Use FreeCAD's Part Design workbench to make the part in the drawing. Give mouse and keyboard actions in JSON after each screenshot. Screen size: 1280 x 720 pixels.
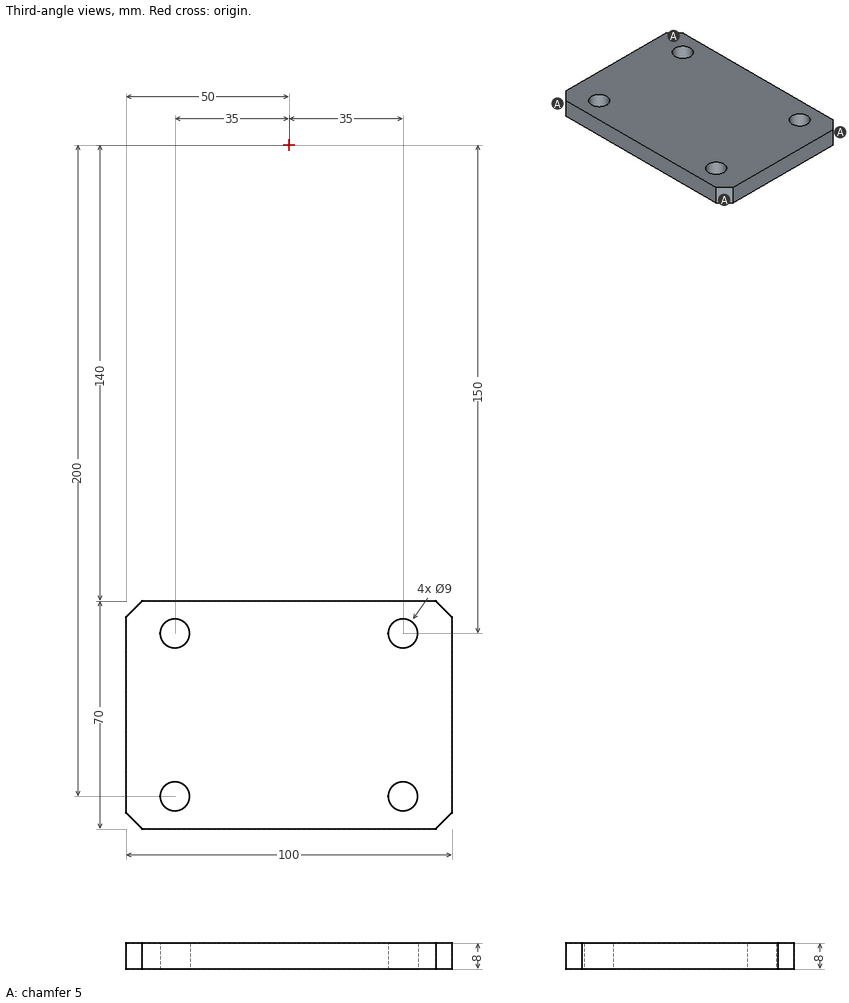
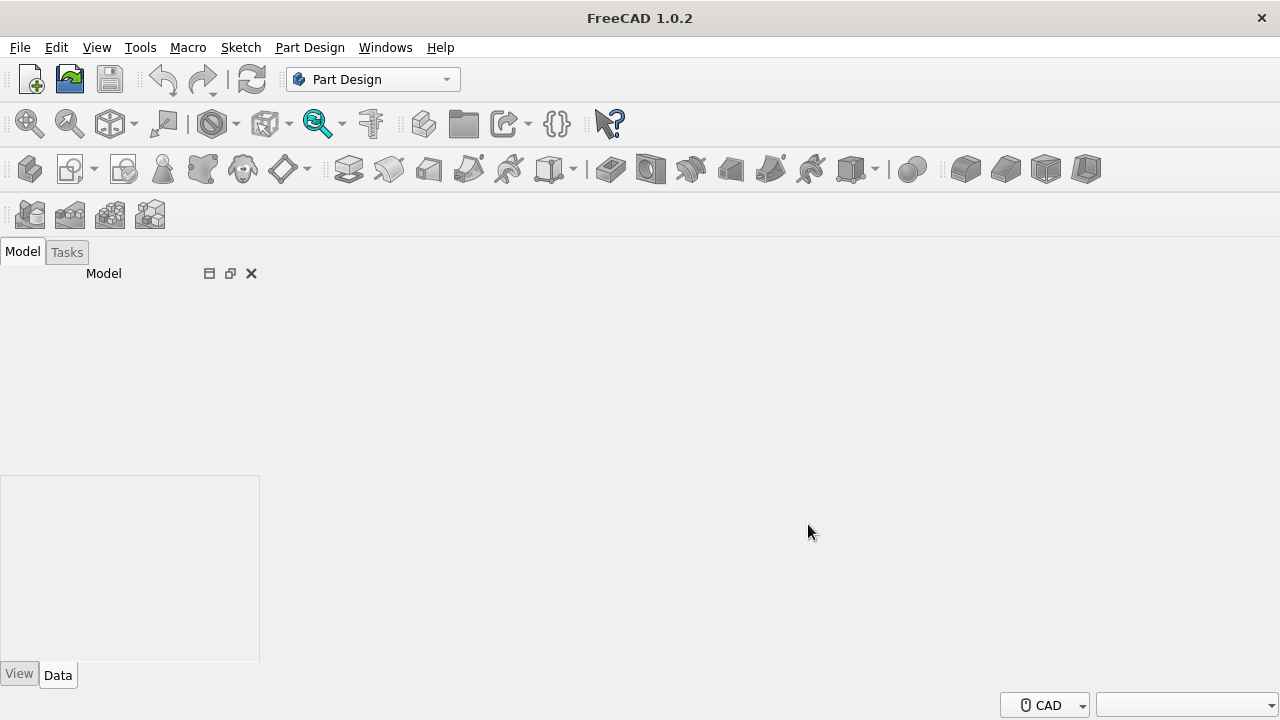
{"action": "left_click", "coordinate": [30, 80]}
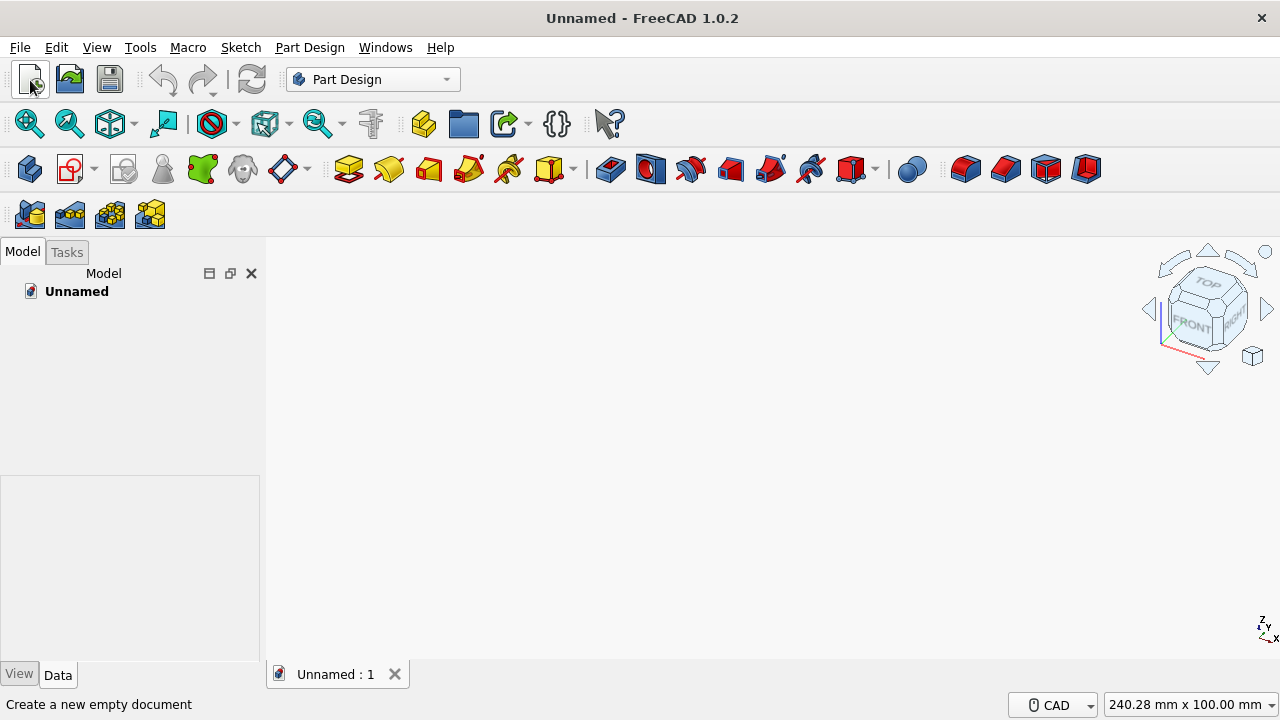
{"action": "left_click", "coordinate": [30, 170]}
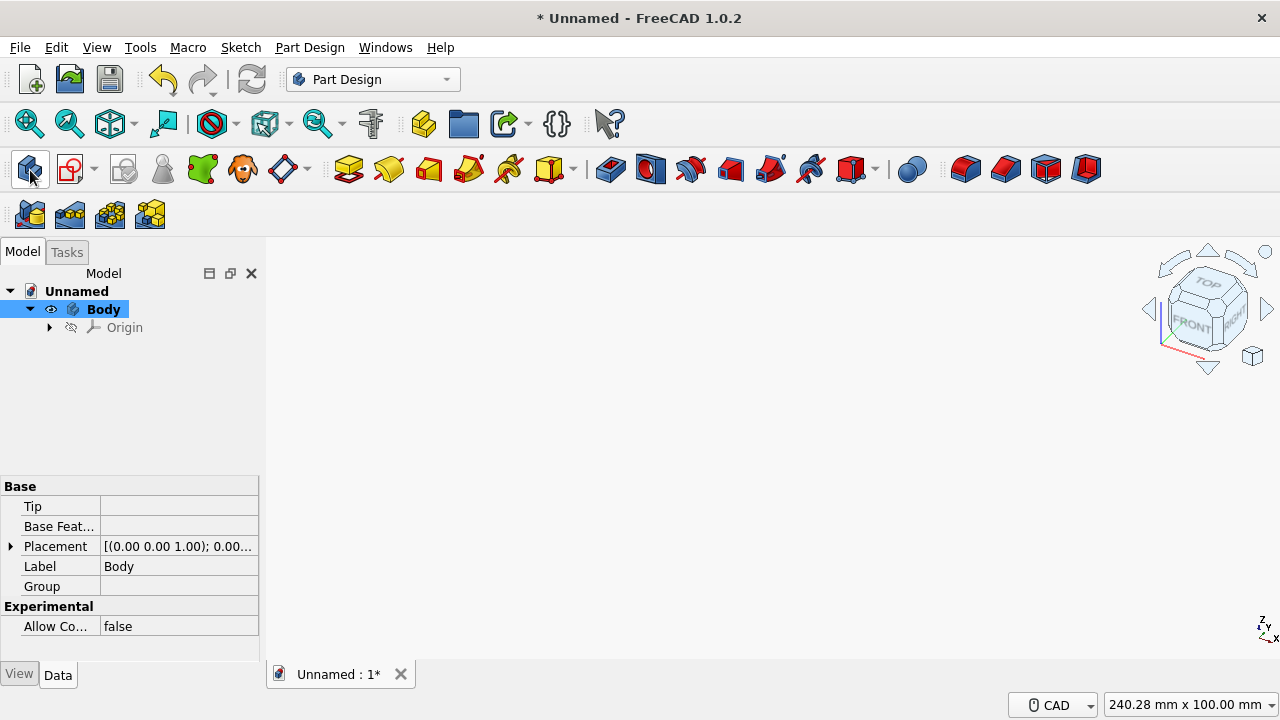
{"action": "left_click", "coordinate": [50, 327]}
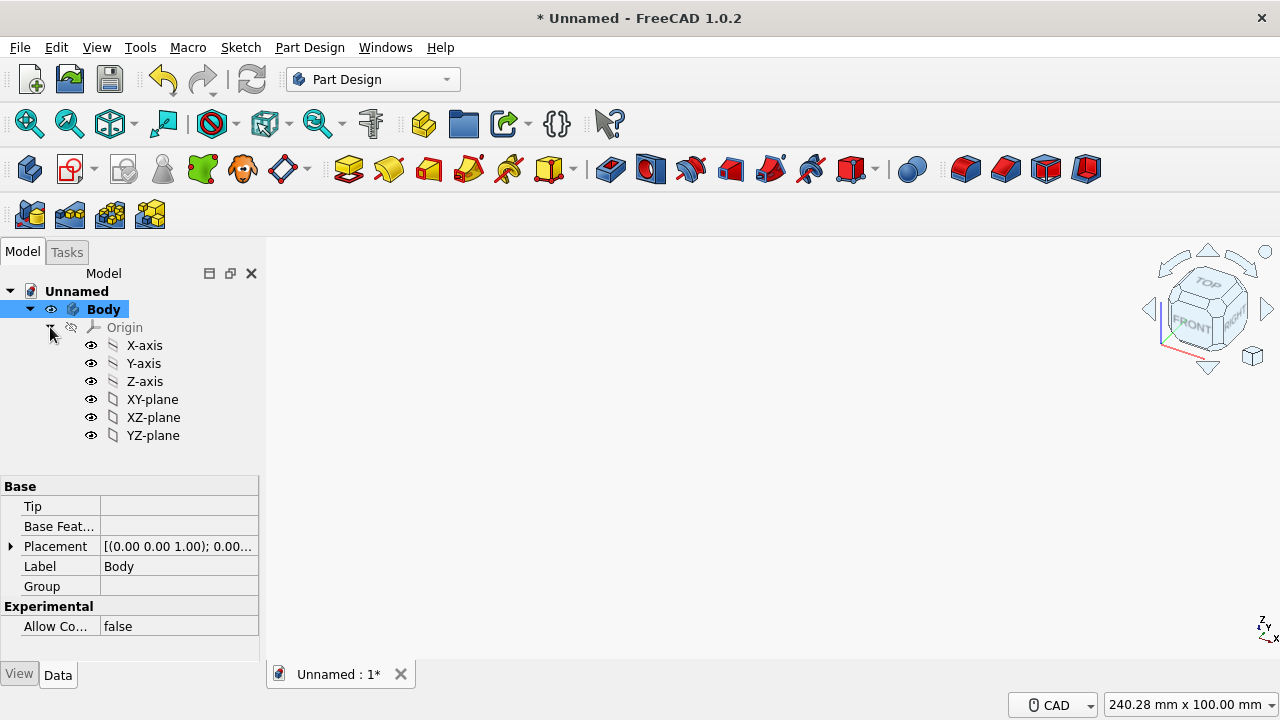
{"action": "left_click", "coordinate": [136, 399]}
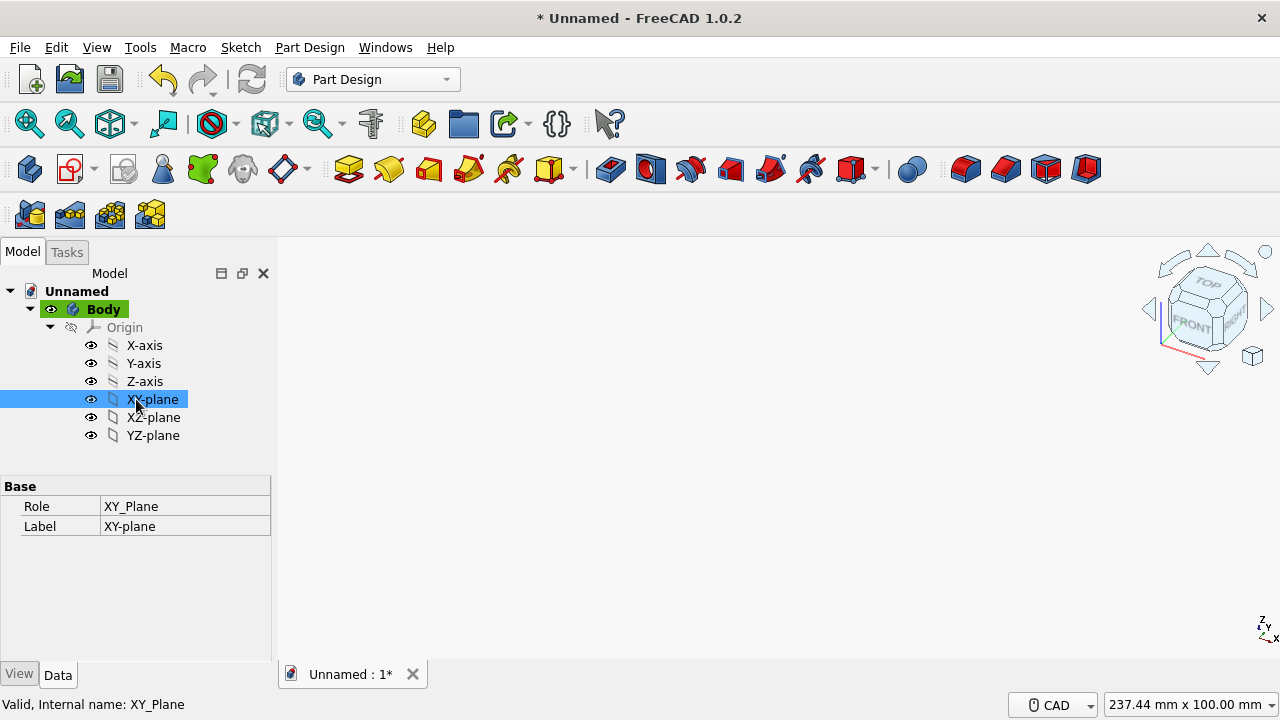
{"action": "left_click", "coordinate": [284, 170]}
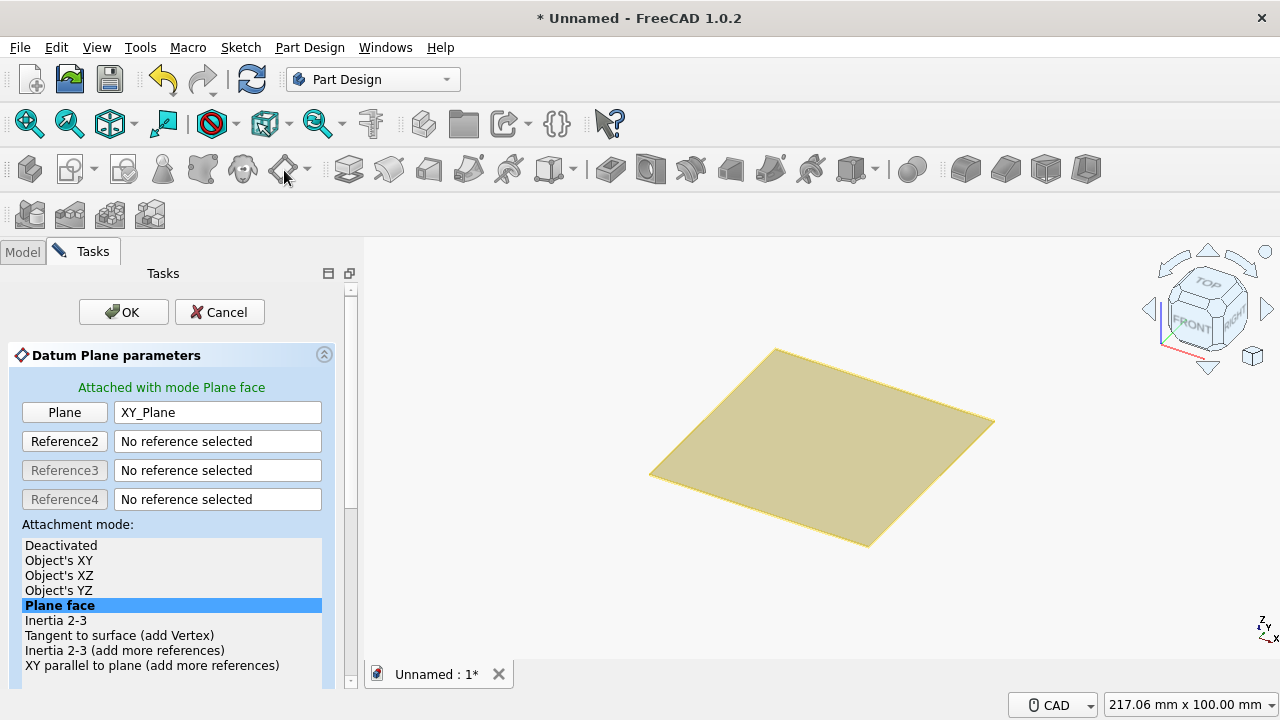
{"action": "scroll", "coordinate": [351, 486], "scroll_direction": "down", "scroll_amount": 4}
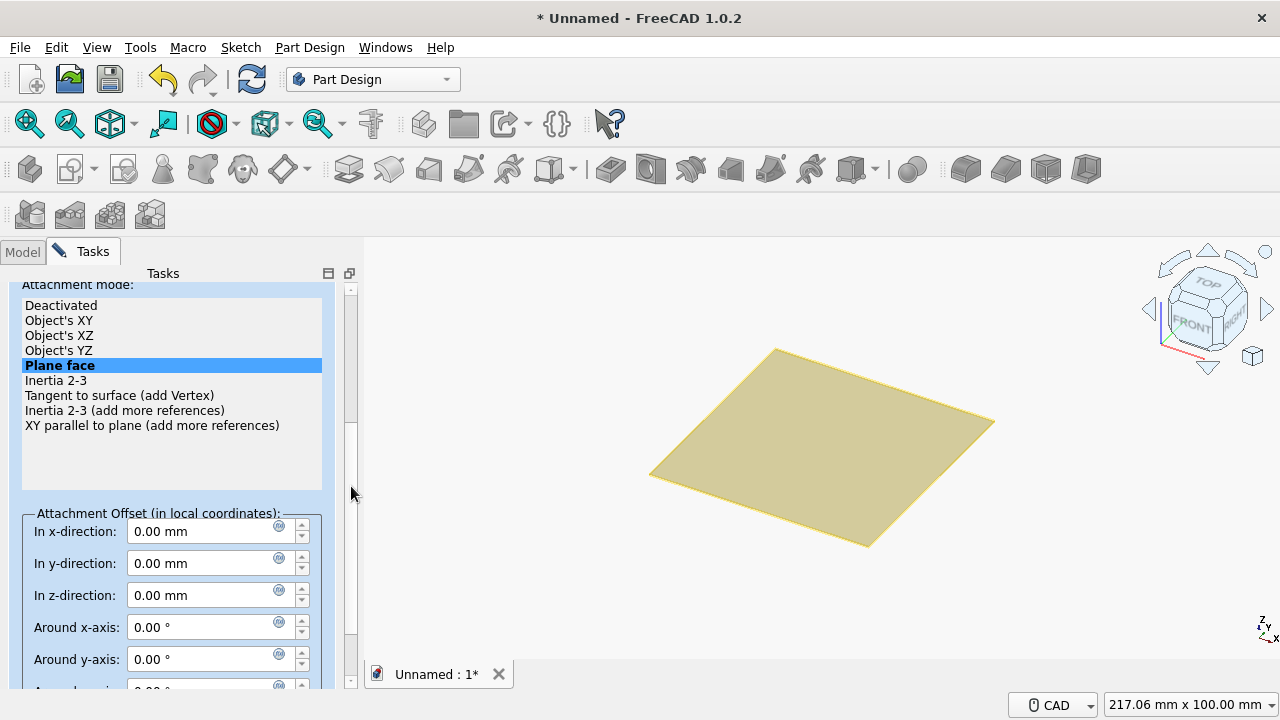
{"action": "triple_click", "coordinate": [210, 595]}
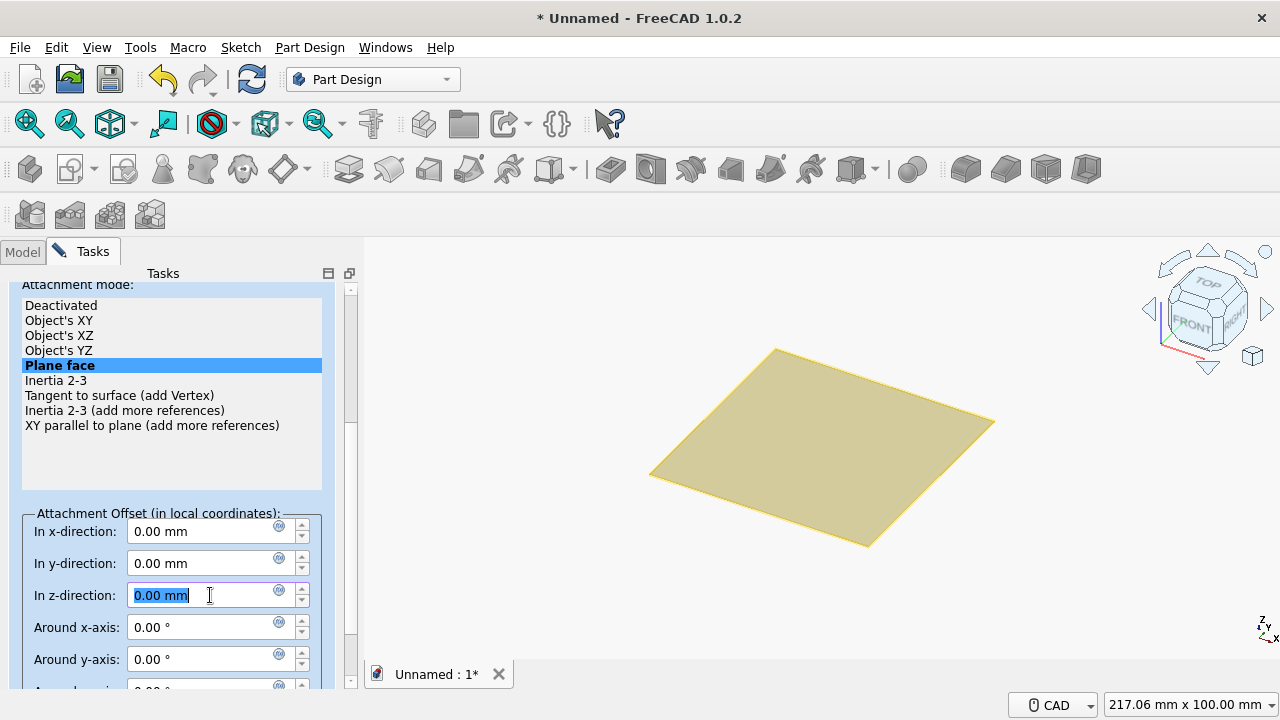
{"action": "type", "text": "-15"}
{"action": "key", "text": "Tab"}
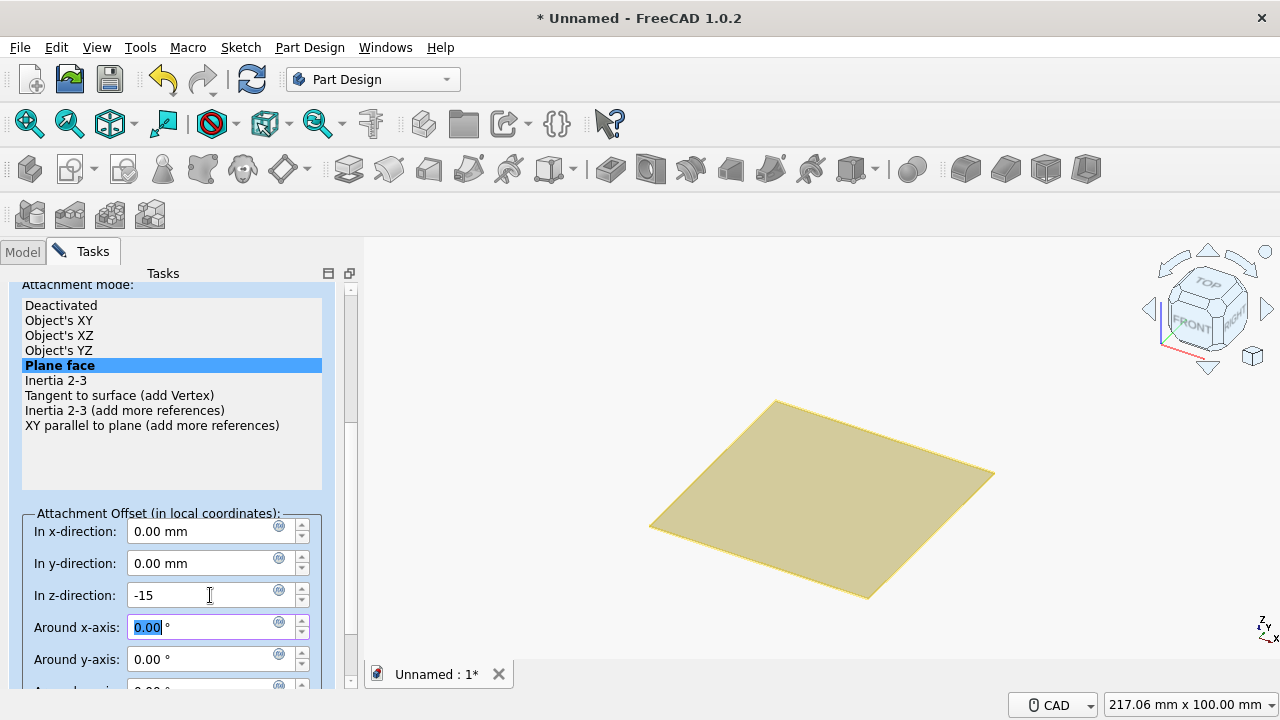
{"action": "scroll", "coordinate": [351, 486], "scroll_direction": "up", "scroll_amount": 5}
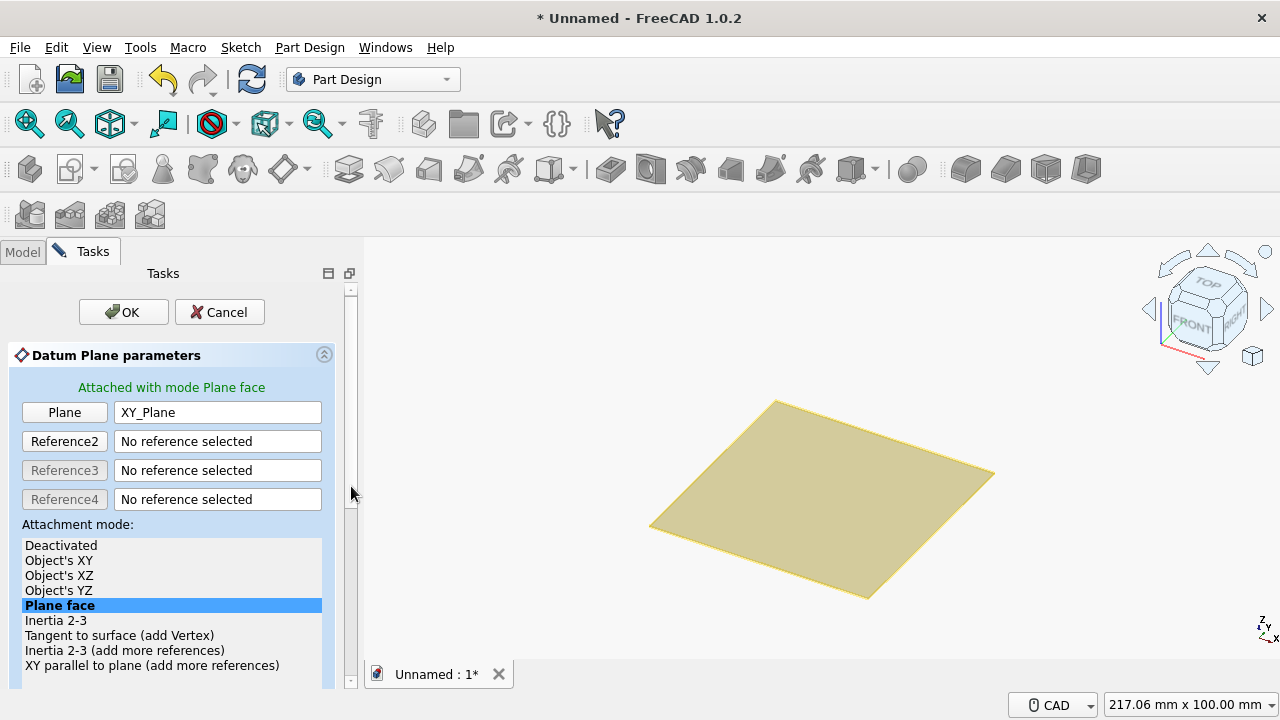
{"action": "left_click", "coordinate": [124, 312]}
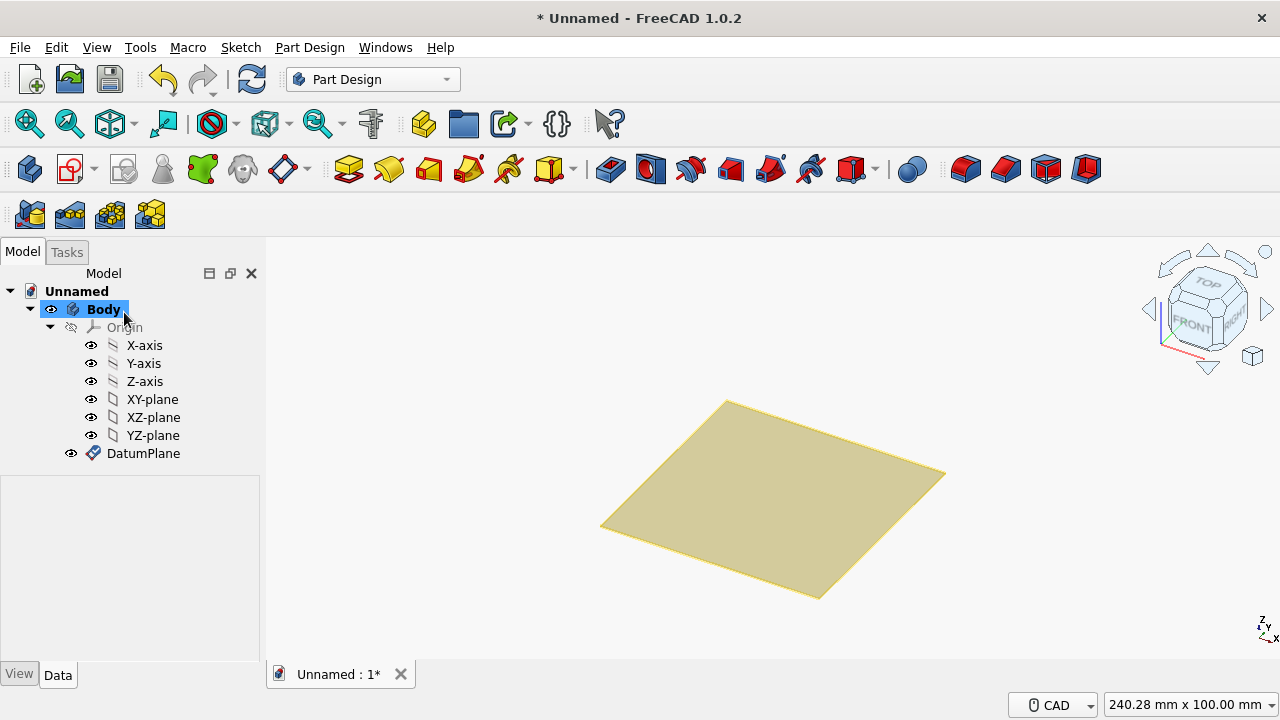
{"action": "left_click", "coordinate": [116, 453]}